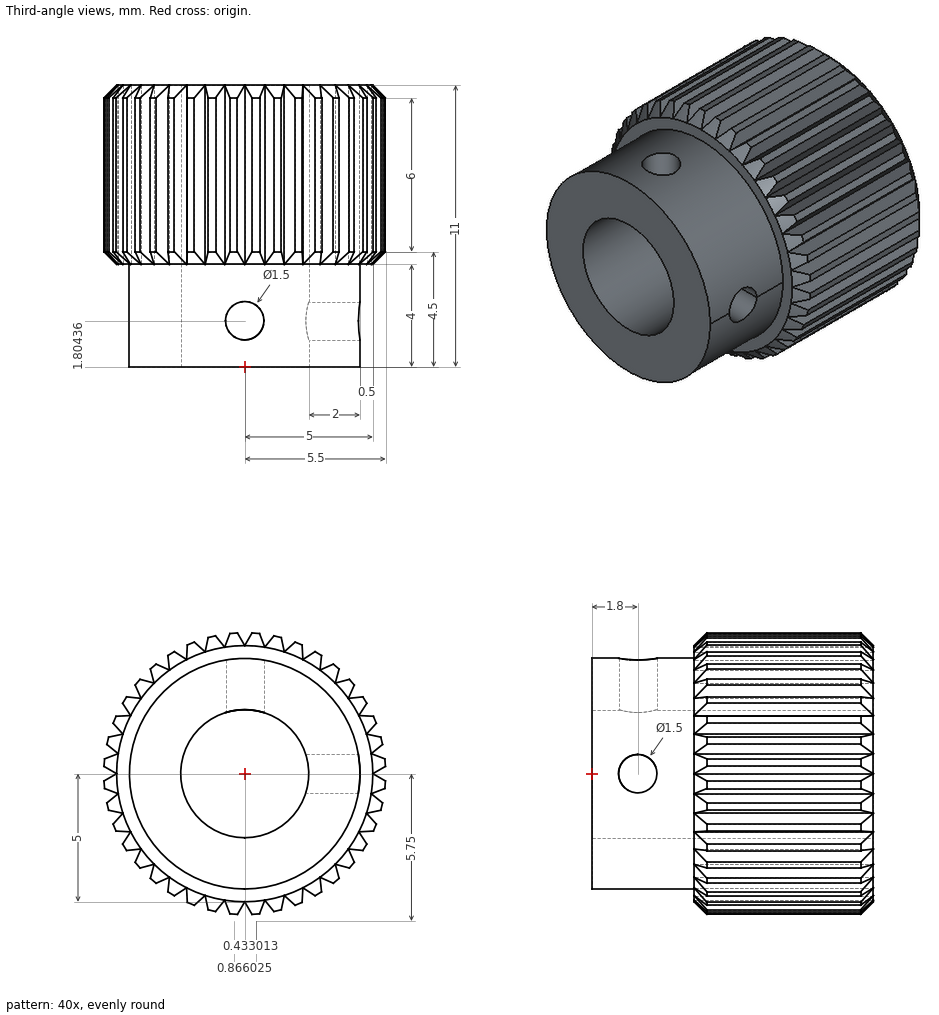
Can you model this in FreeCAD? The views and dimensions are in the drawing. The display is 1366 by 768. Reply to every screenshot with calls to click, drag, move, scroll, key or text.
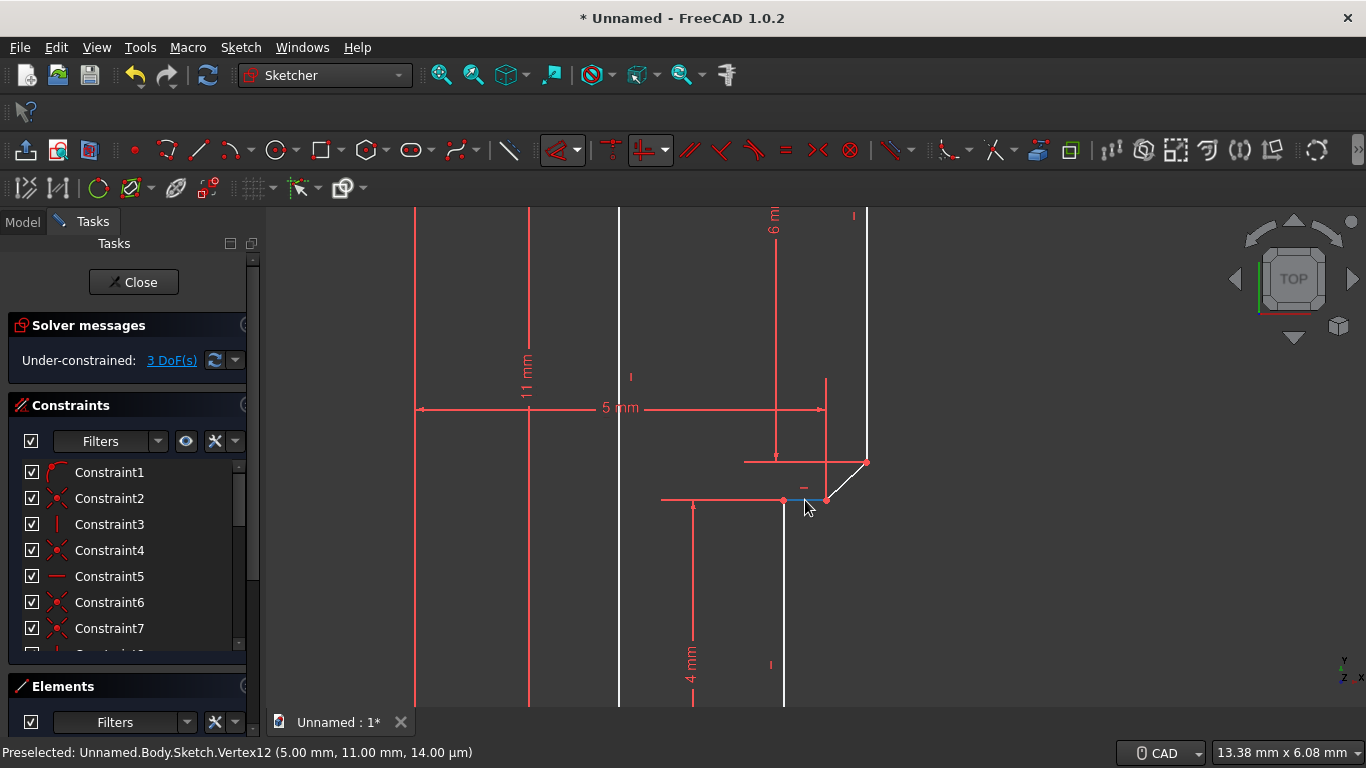
click(805, 500)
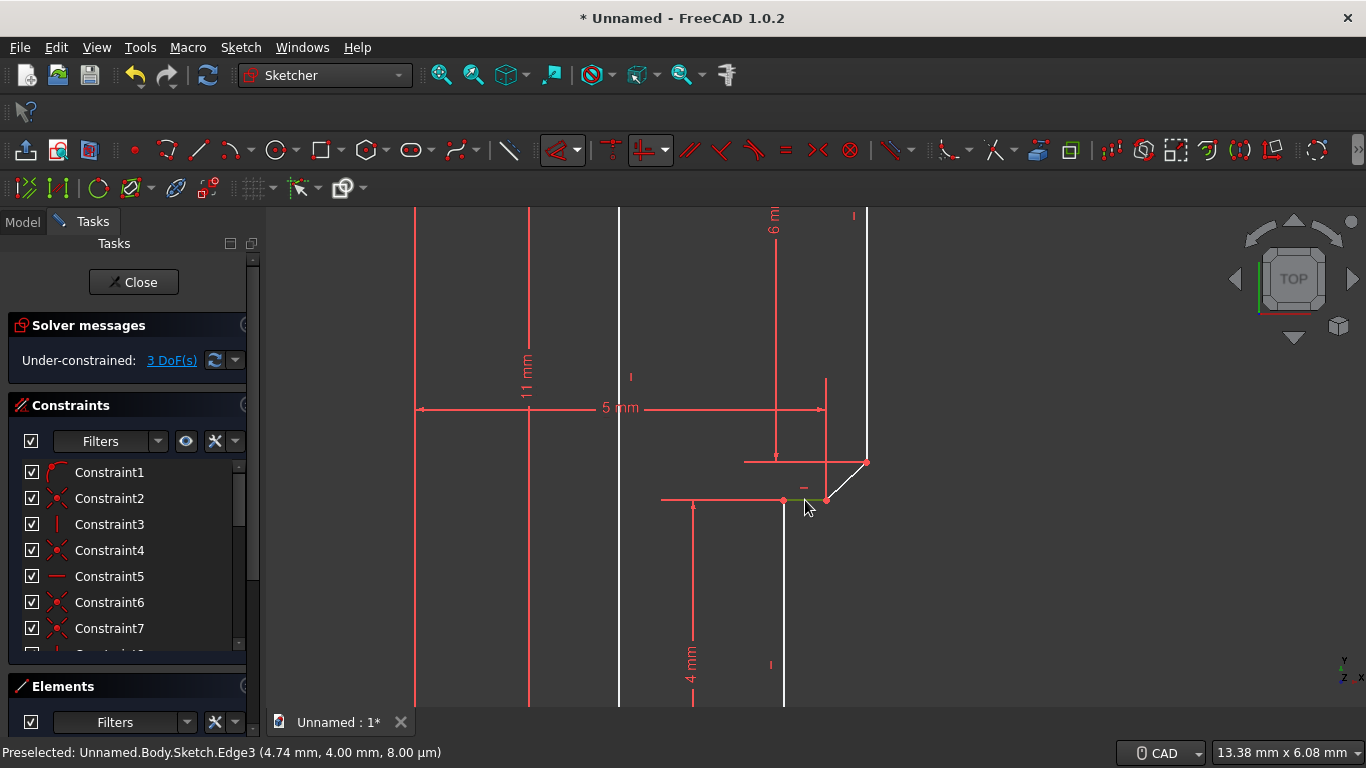
key(l)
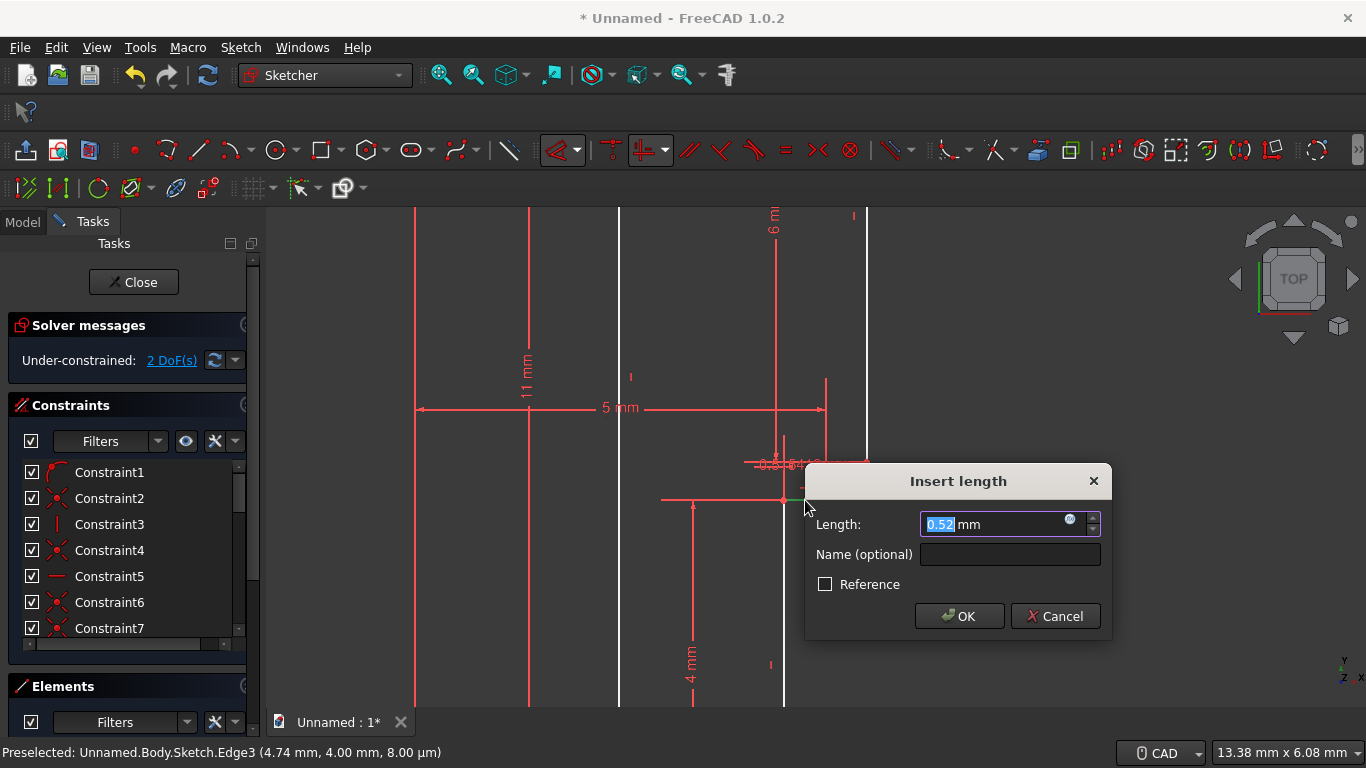
text(0.5)
key(Return)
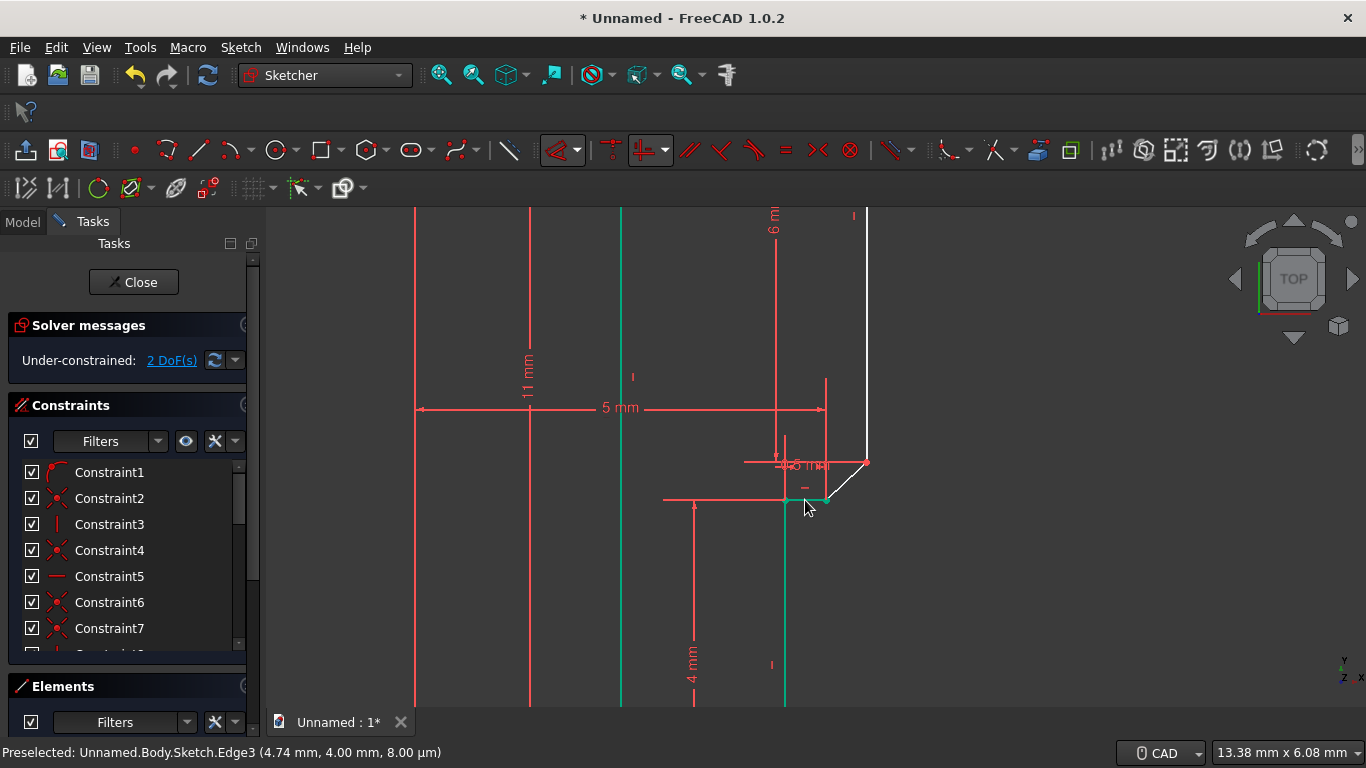
click(867, 462)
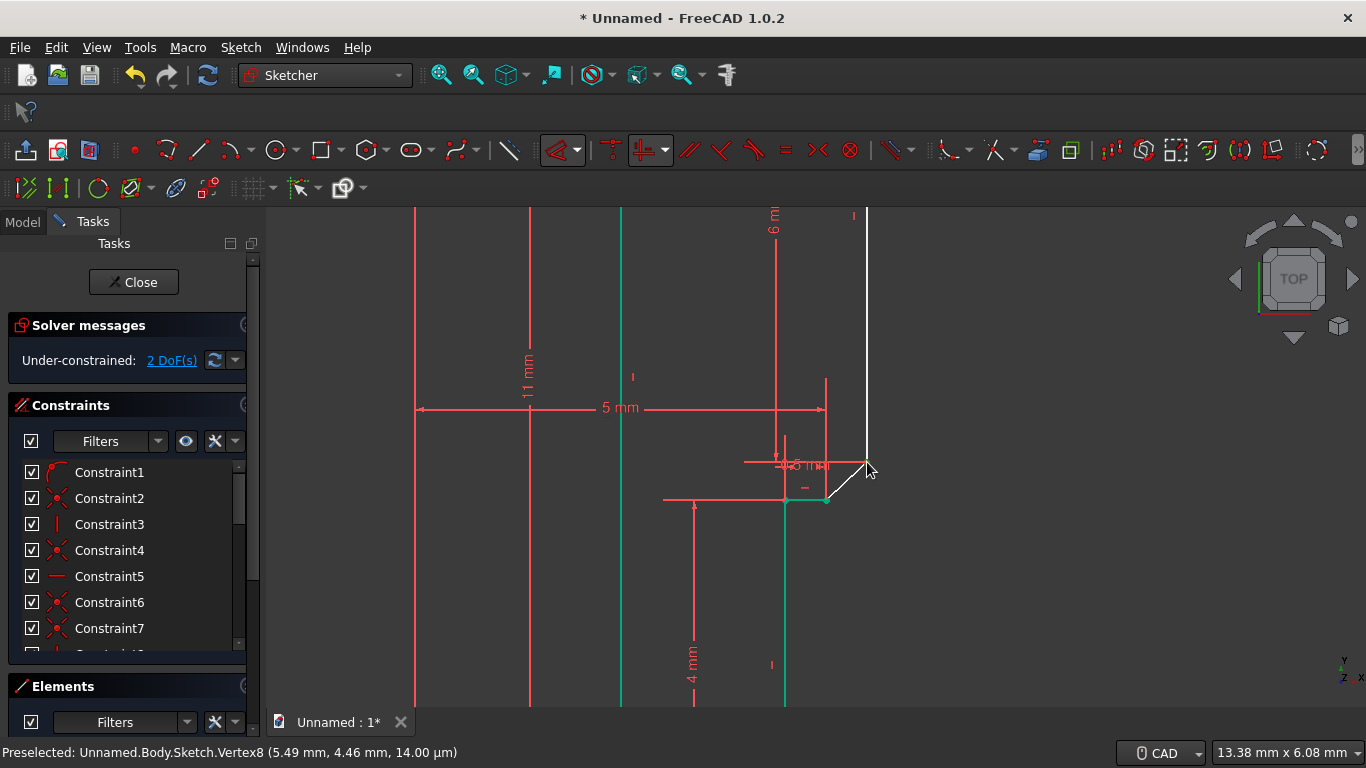
key(l)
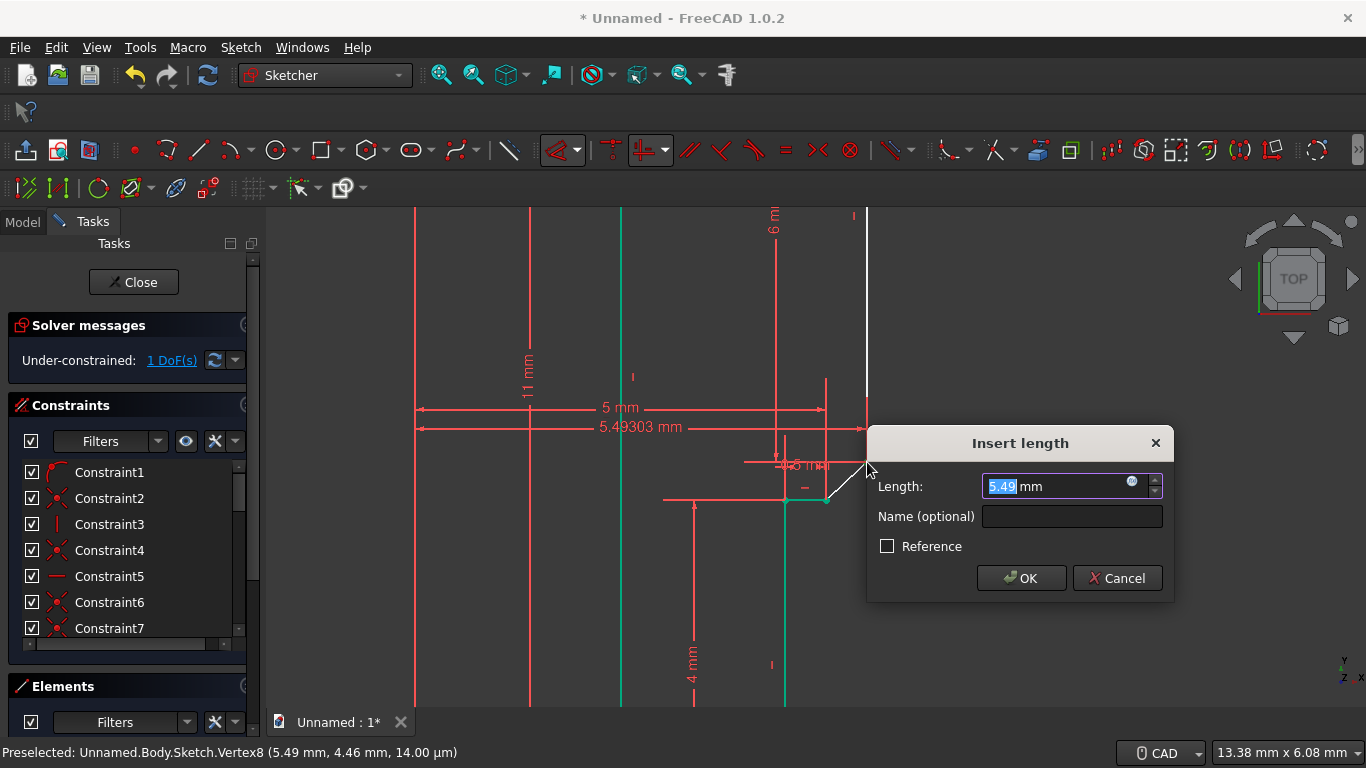
text(5.5)
key(Return)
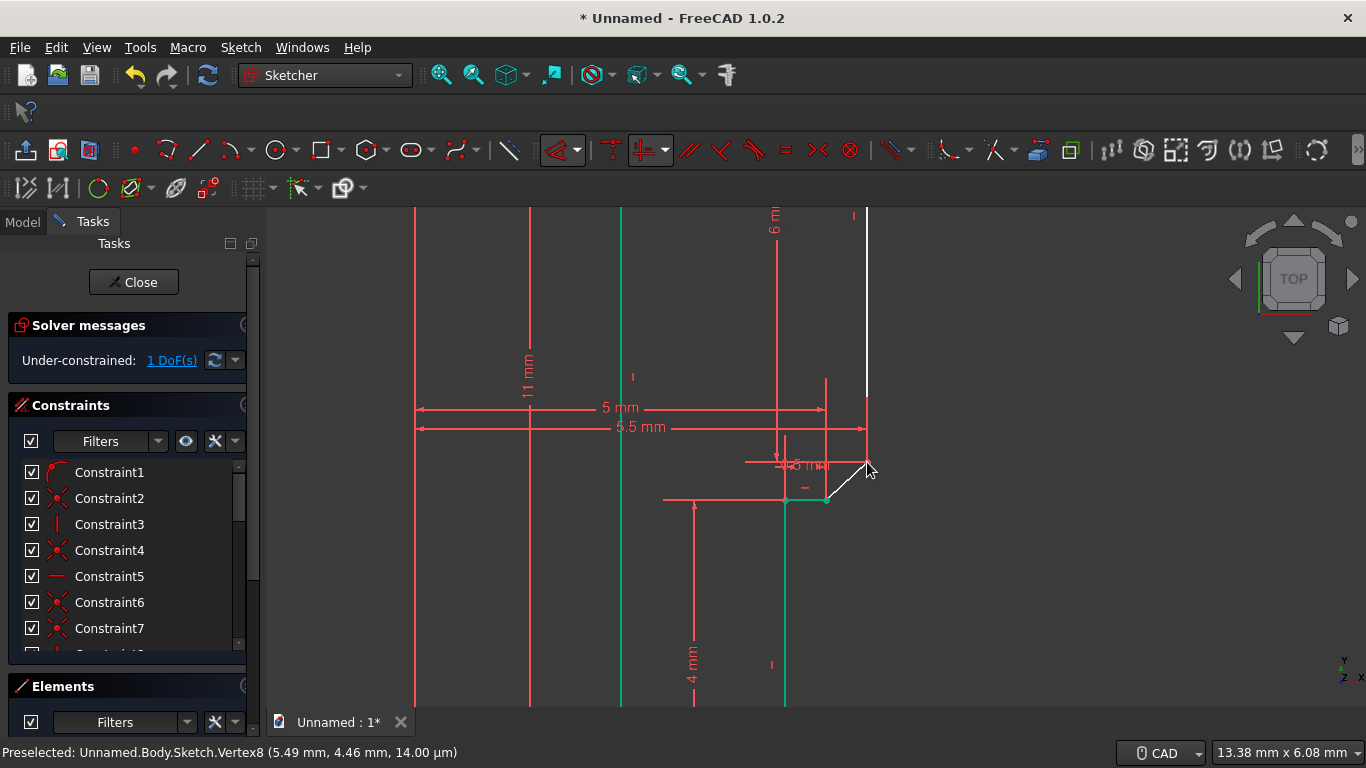
click(867, 462)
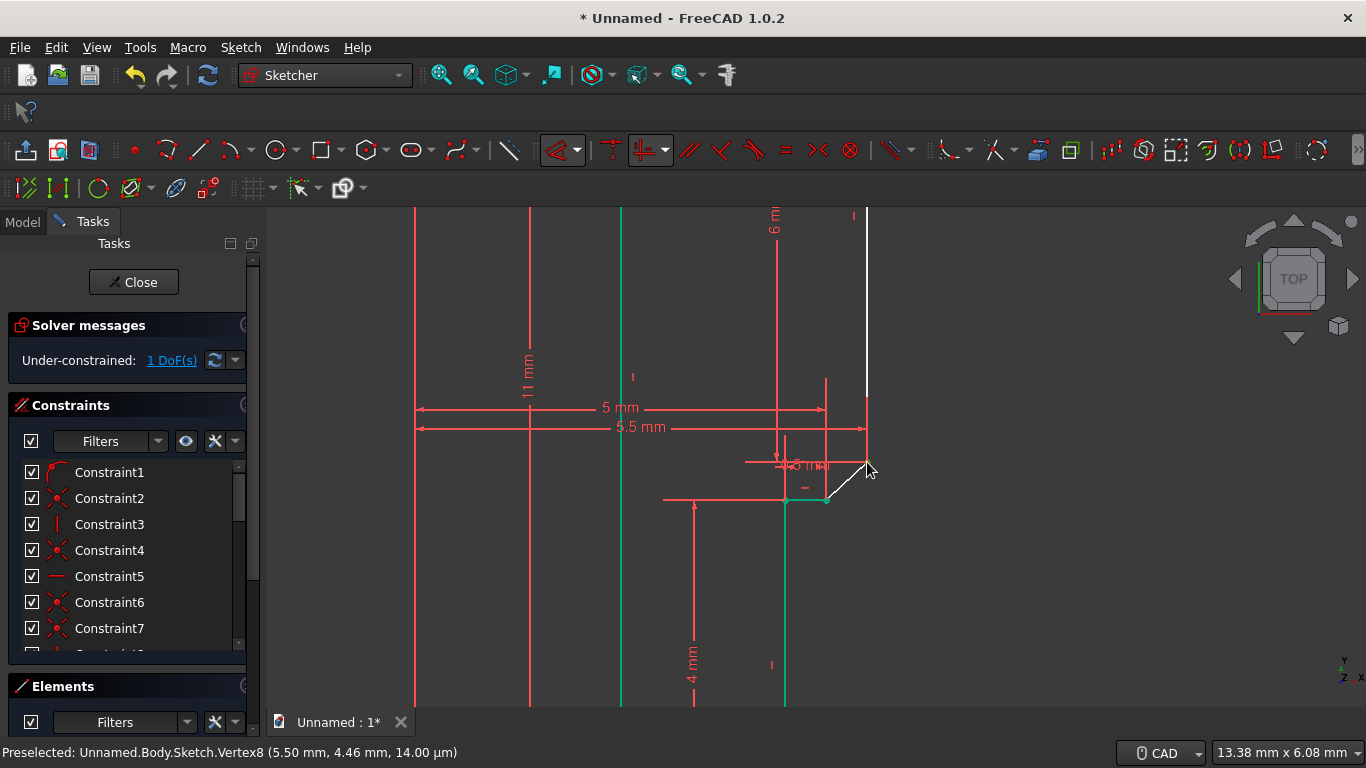
key(i)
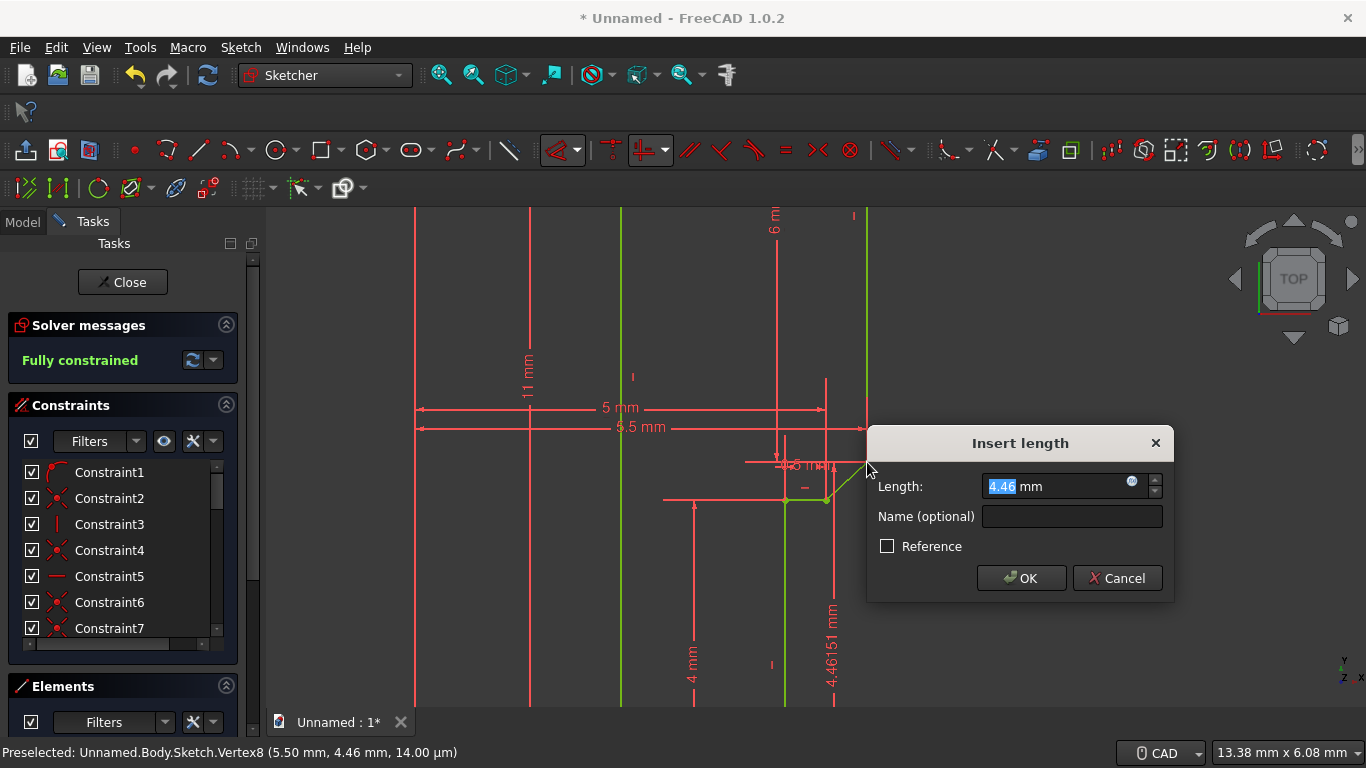
text(4.5)
key(Return)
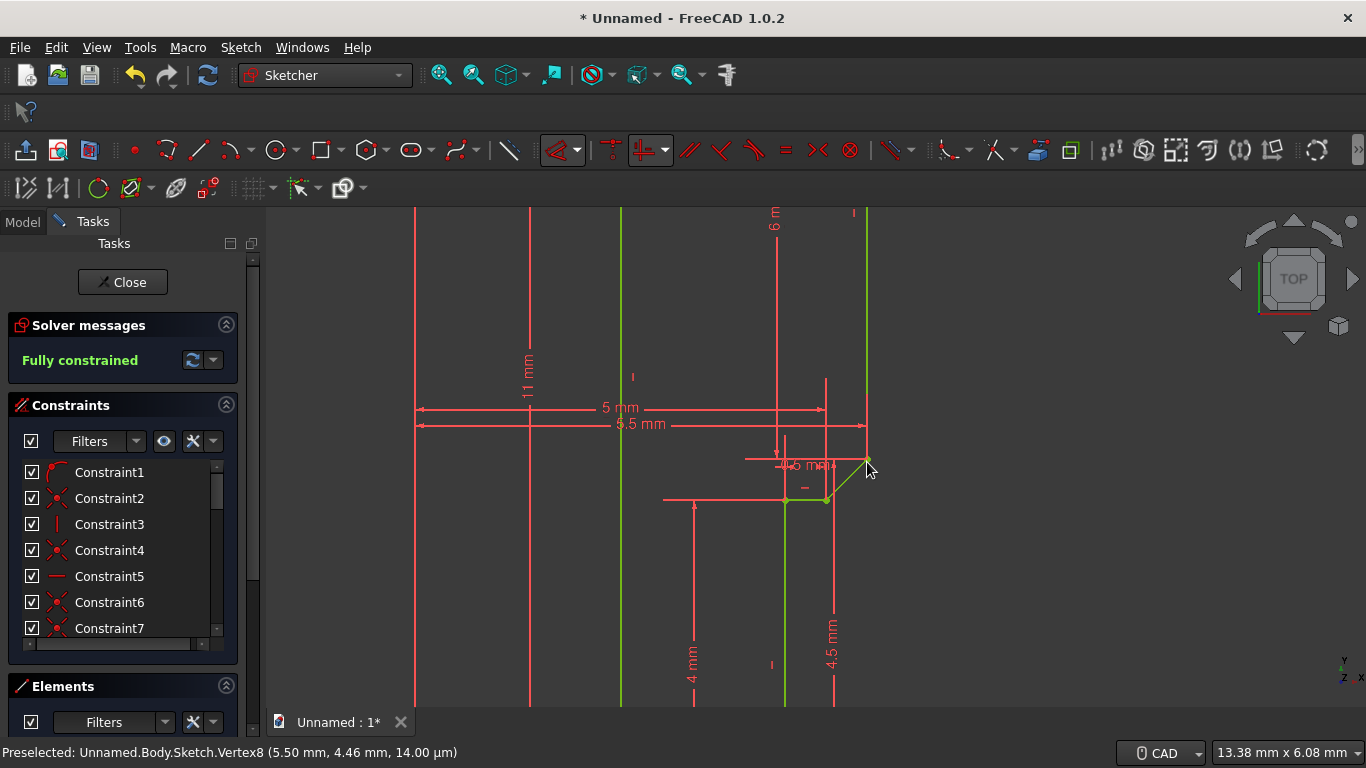
click(123, 282)